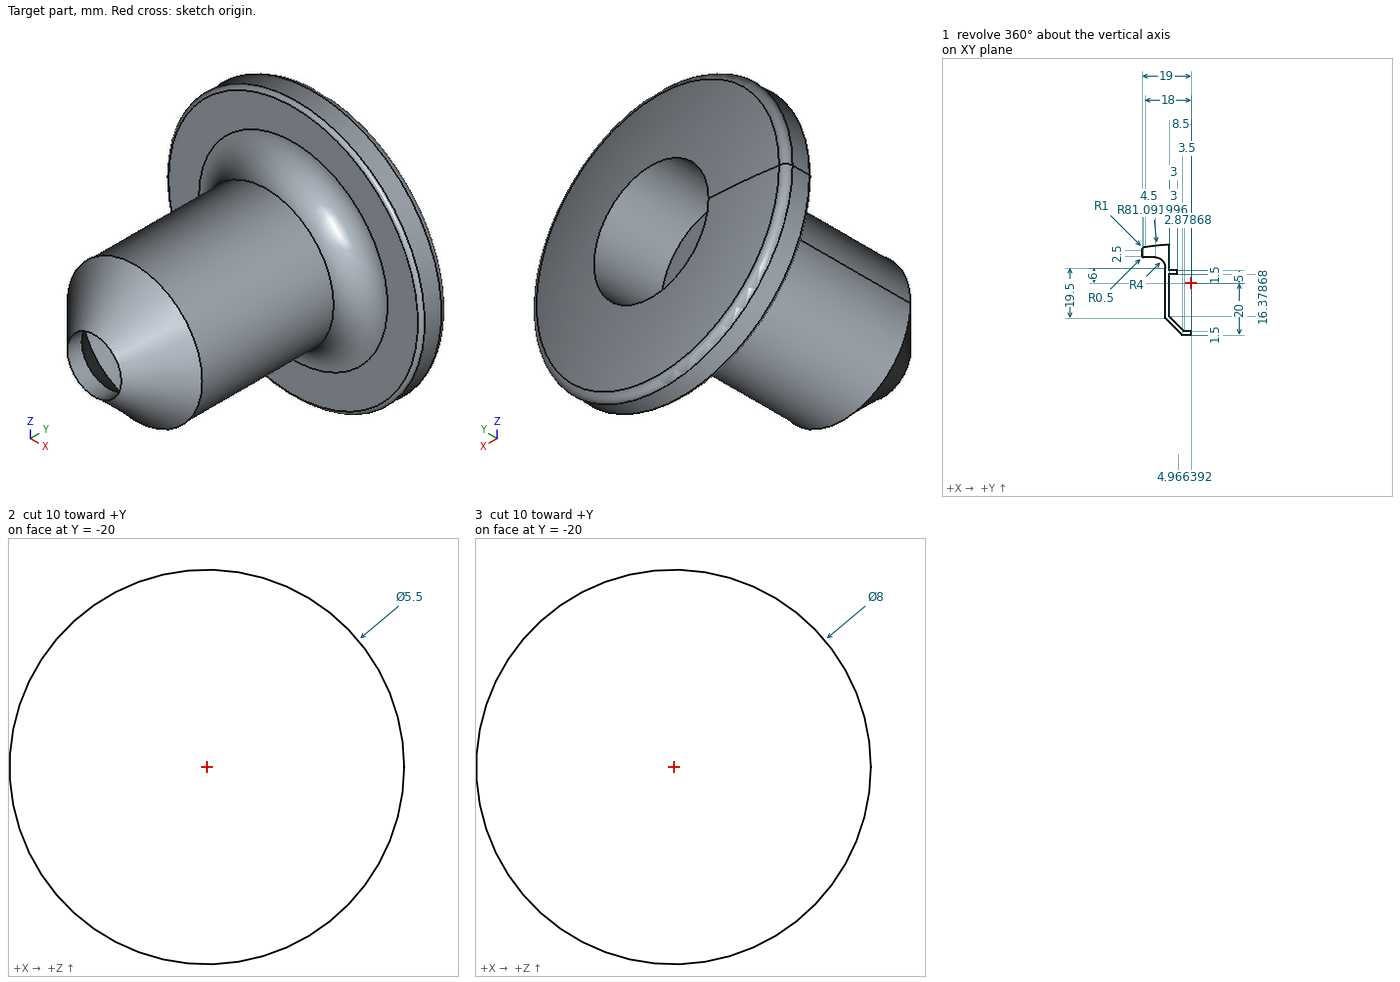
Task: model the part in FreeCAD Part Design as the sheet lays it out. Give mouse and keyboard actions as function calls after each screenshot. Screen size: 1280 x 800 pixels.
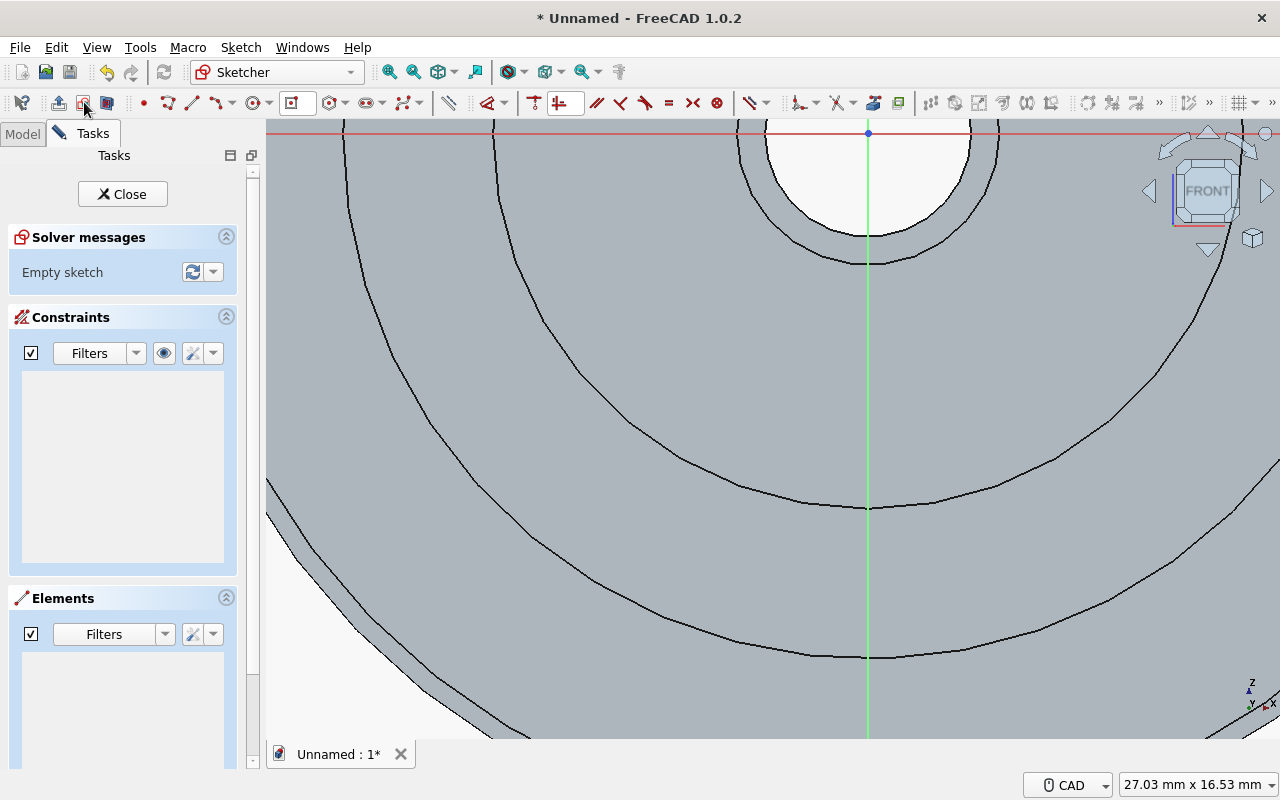
scroll(372, 711, down, 2)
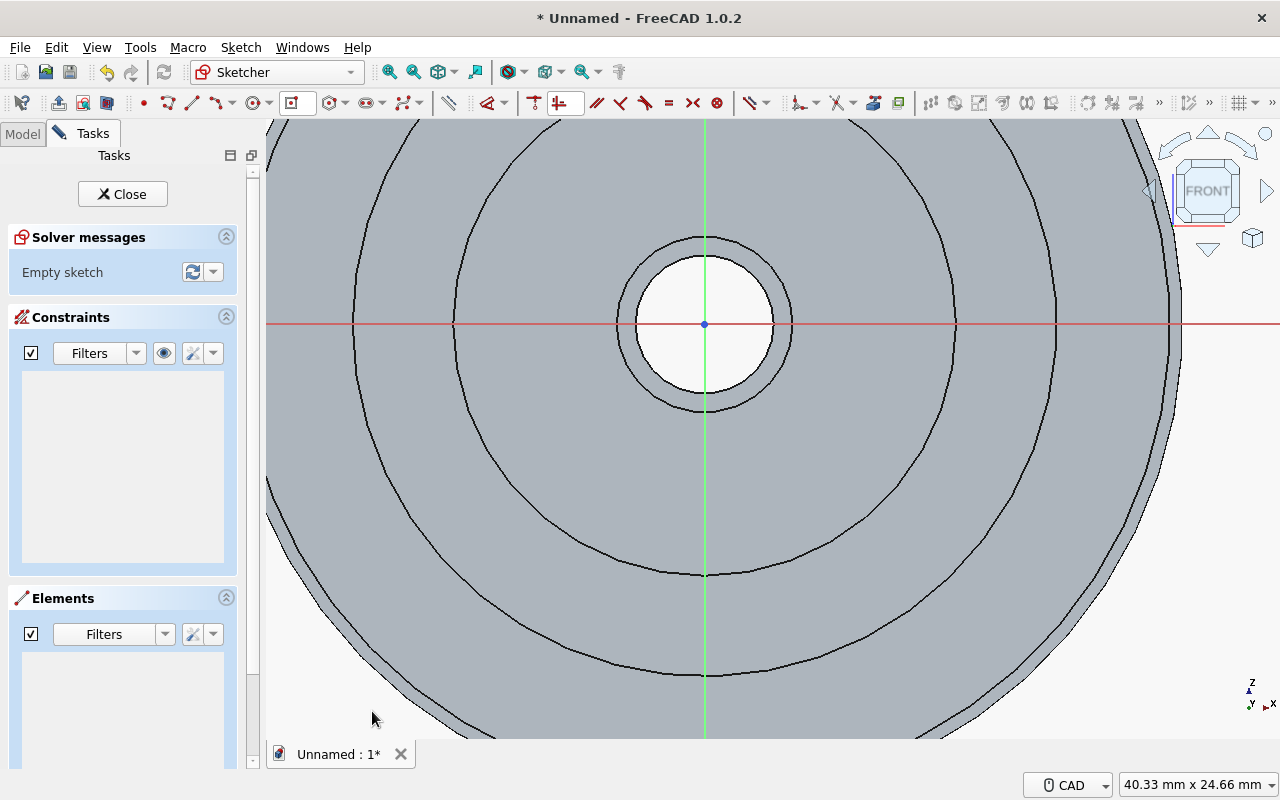
scroll(705, 197, up, 3)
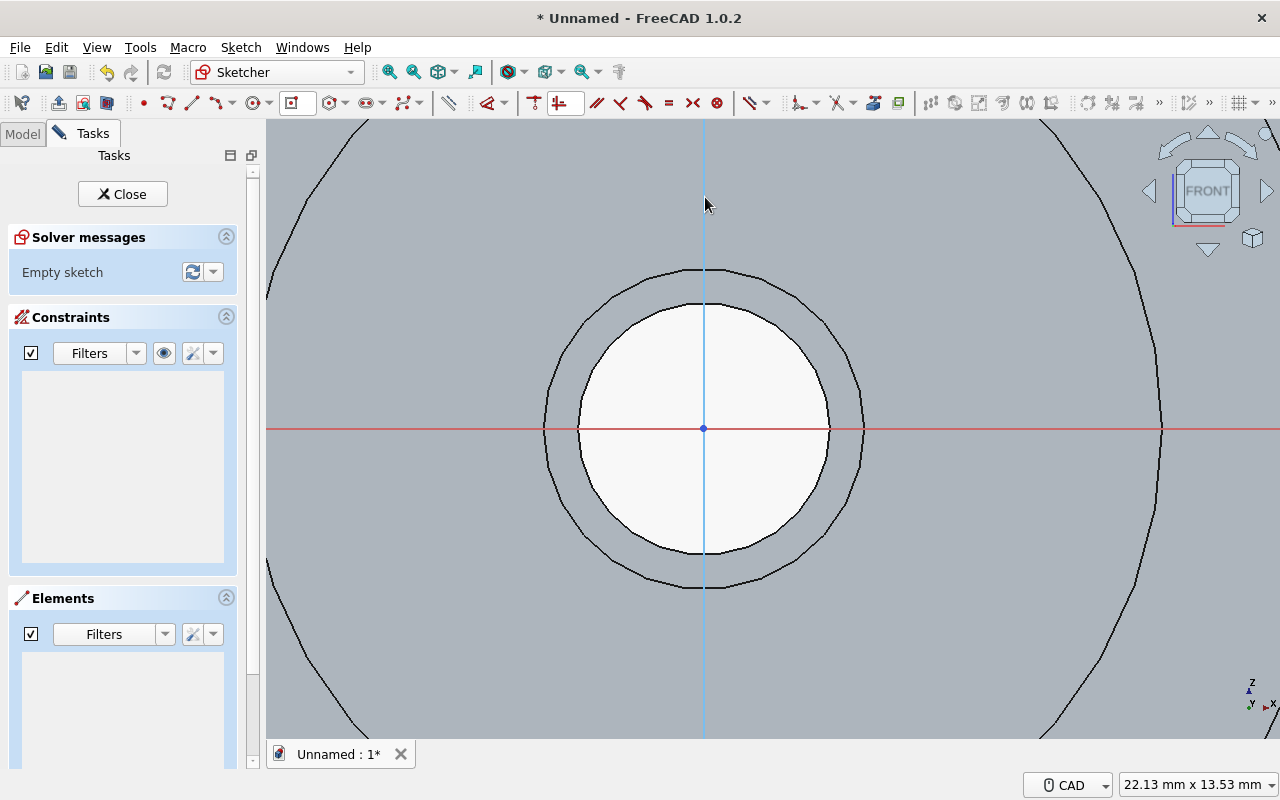
click(254, 104)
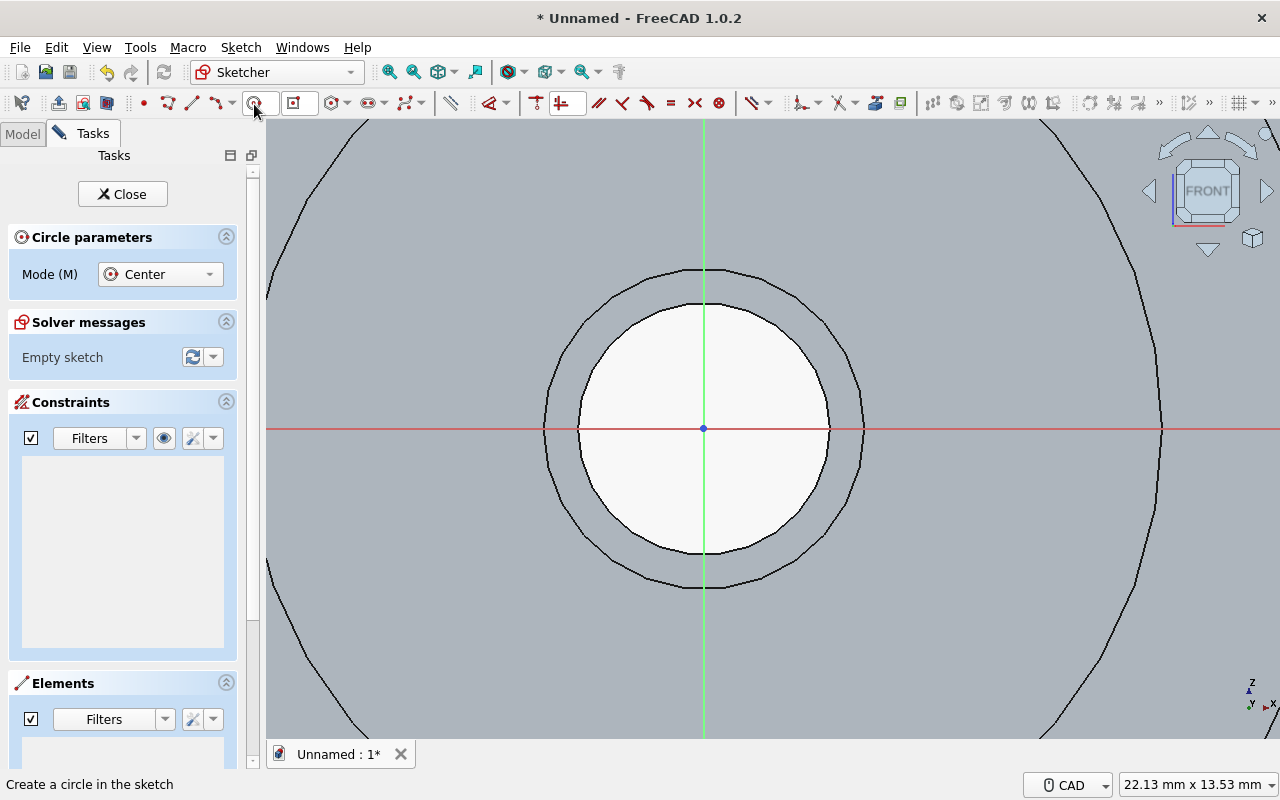
click(704, 429)
move(834, 299)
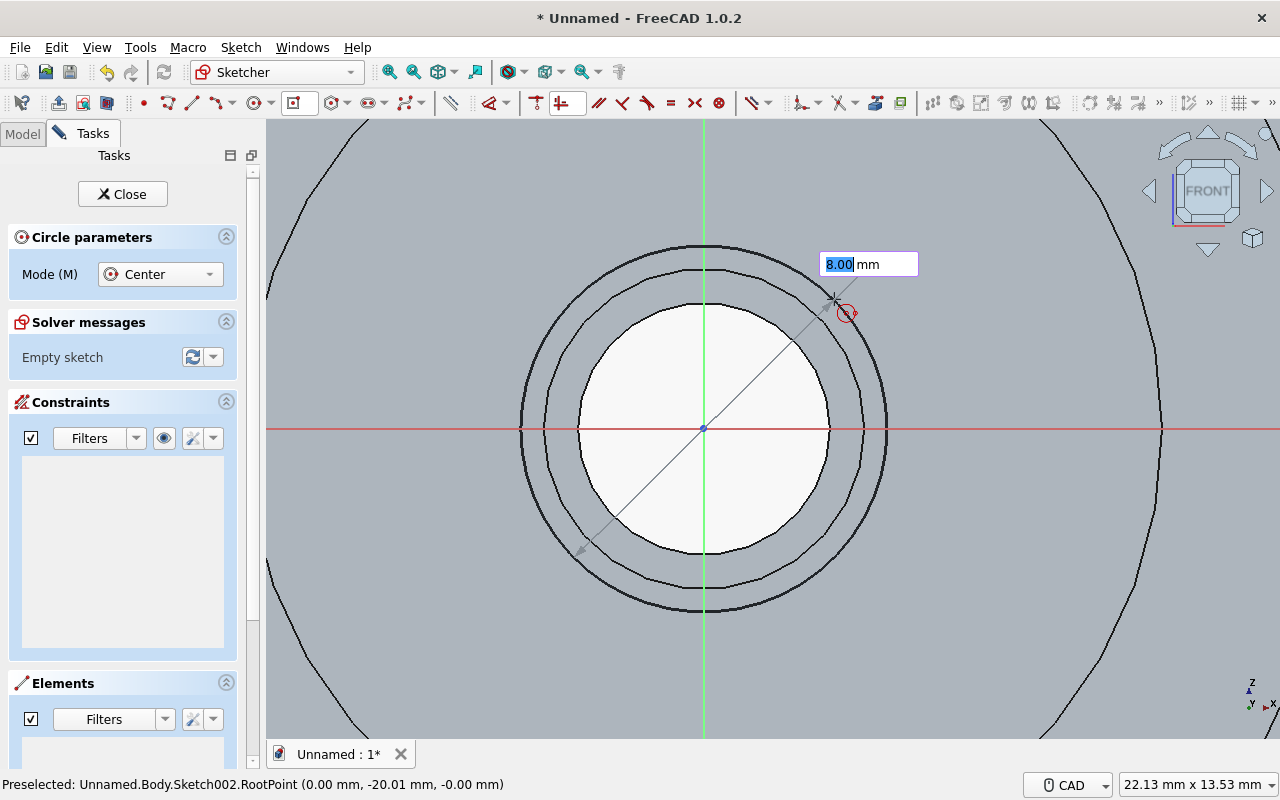
text(8)
key(Return)
key(Escape)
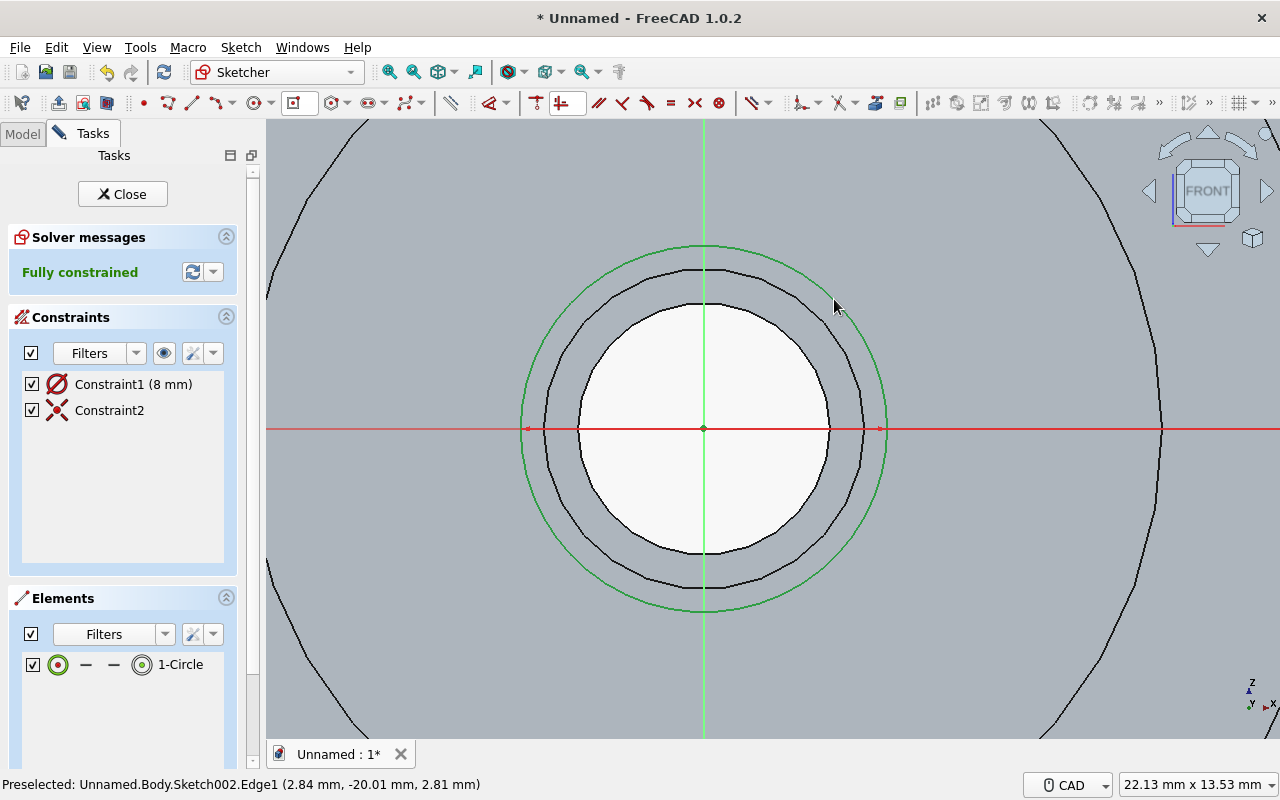
click(123, 194)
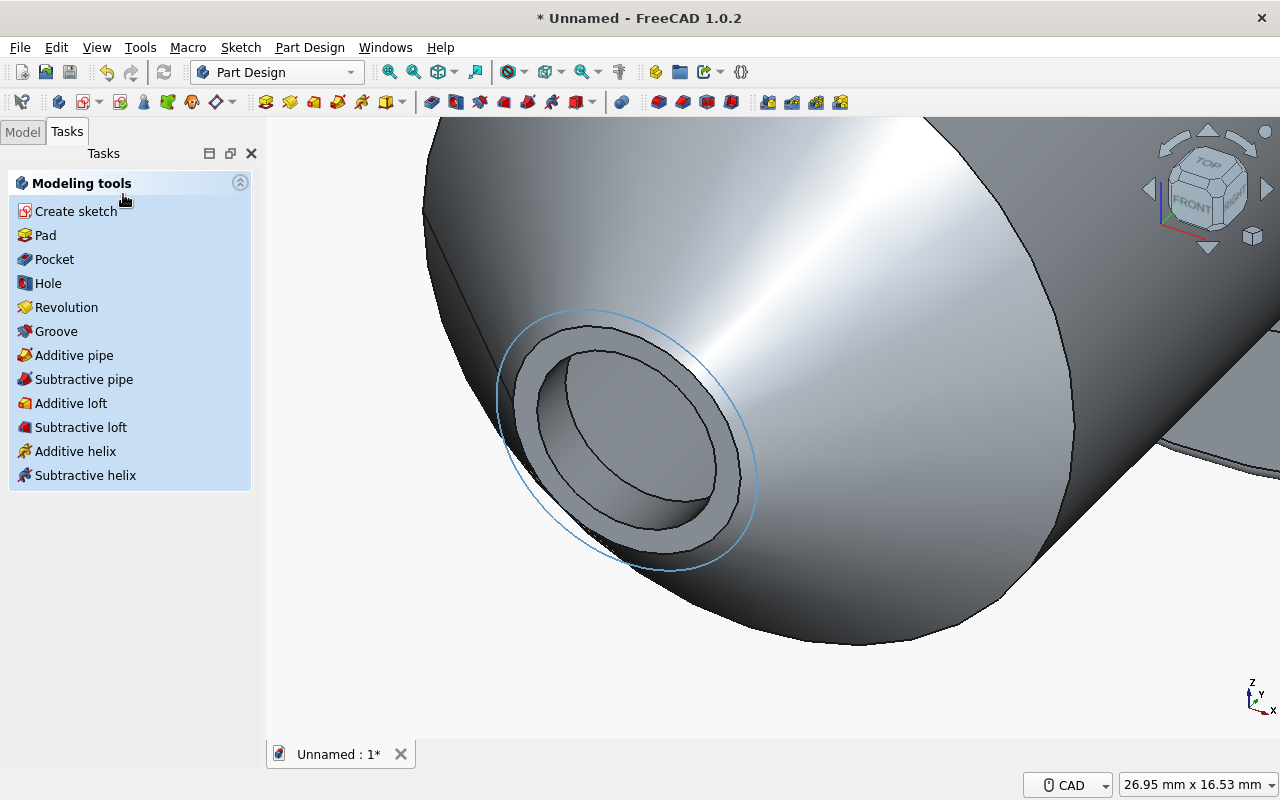
click(432, 102)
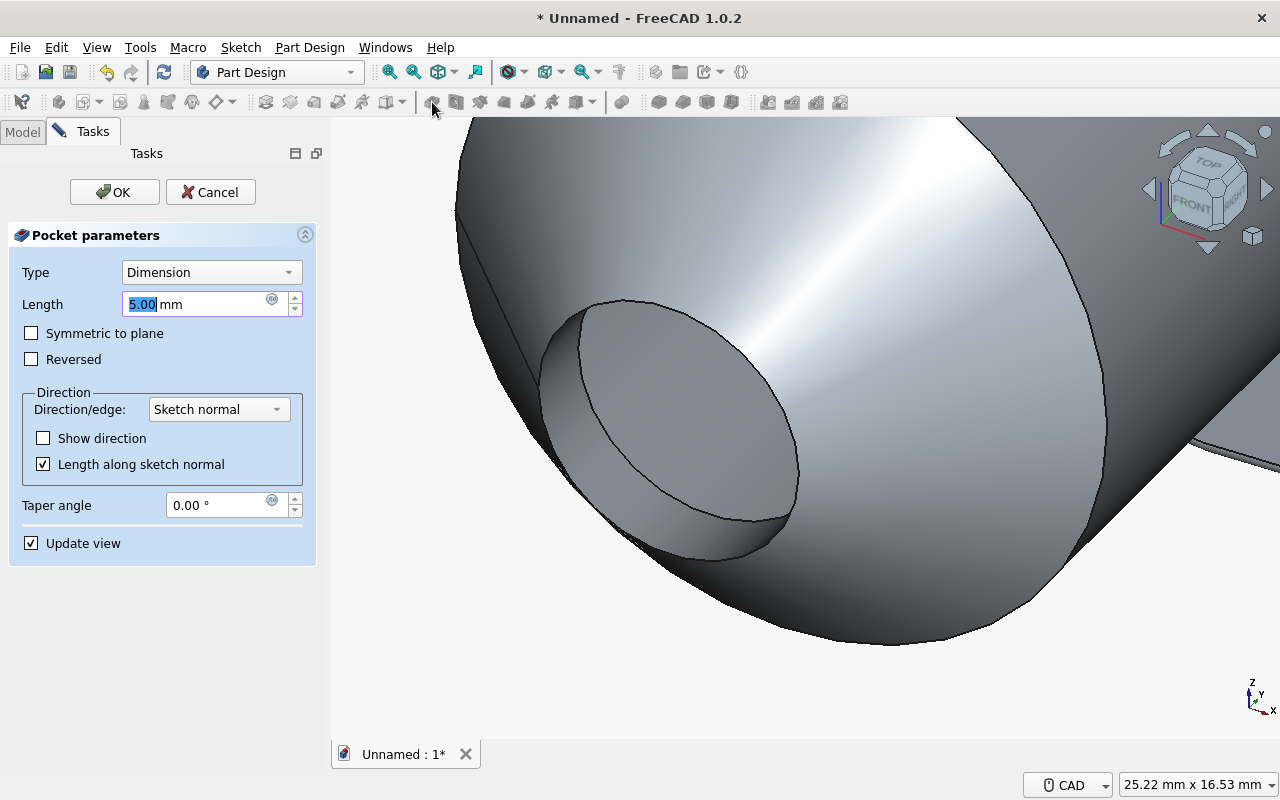
text(10)
key(Tab)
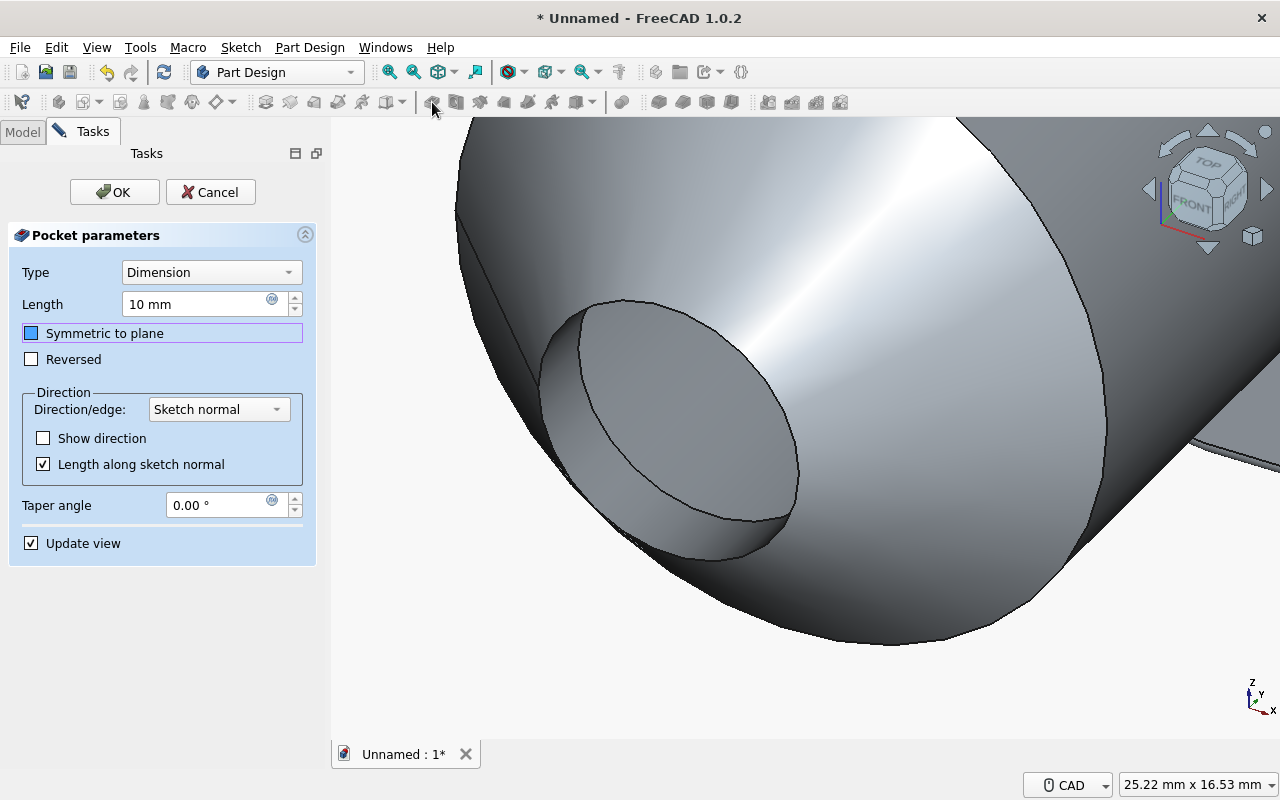
click(115, 192)